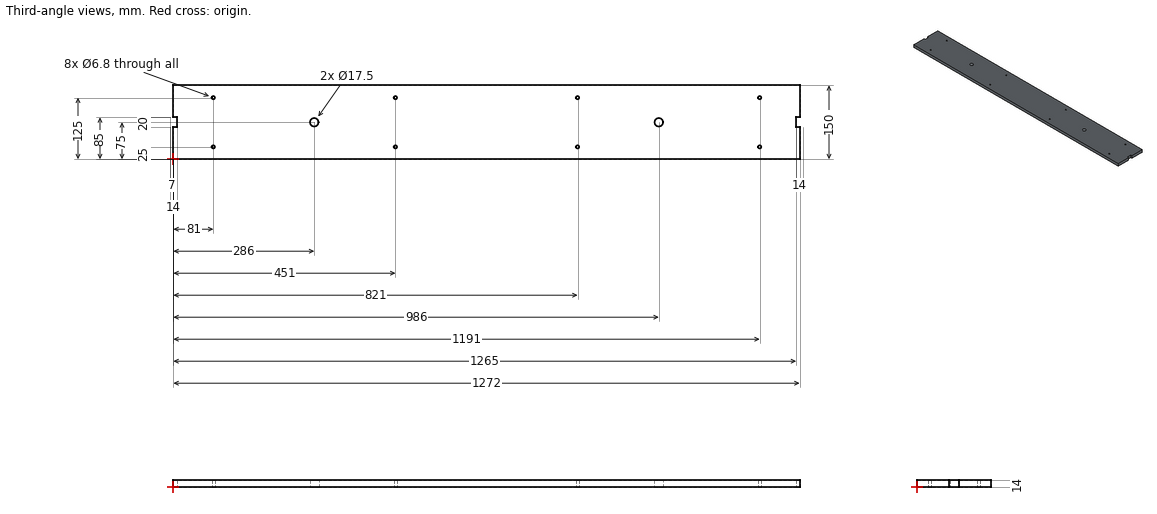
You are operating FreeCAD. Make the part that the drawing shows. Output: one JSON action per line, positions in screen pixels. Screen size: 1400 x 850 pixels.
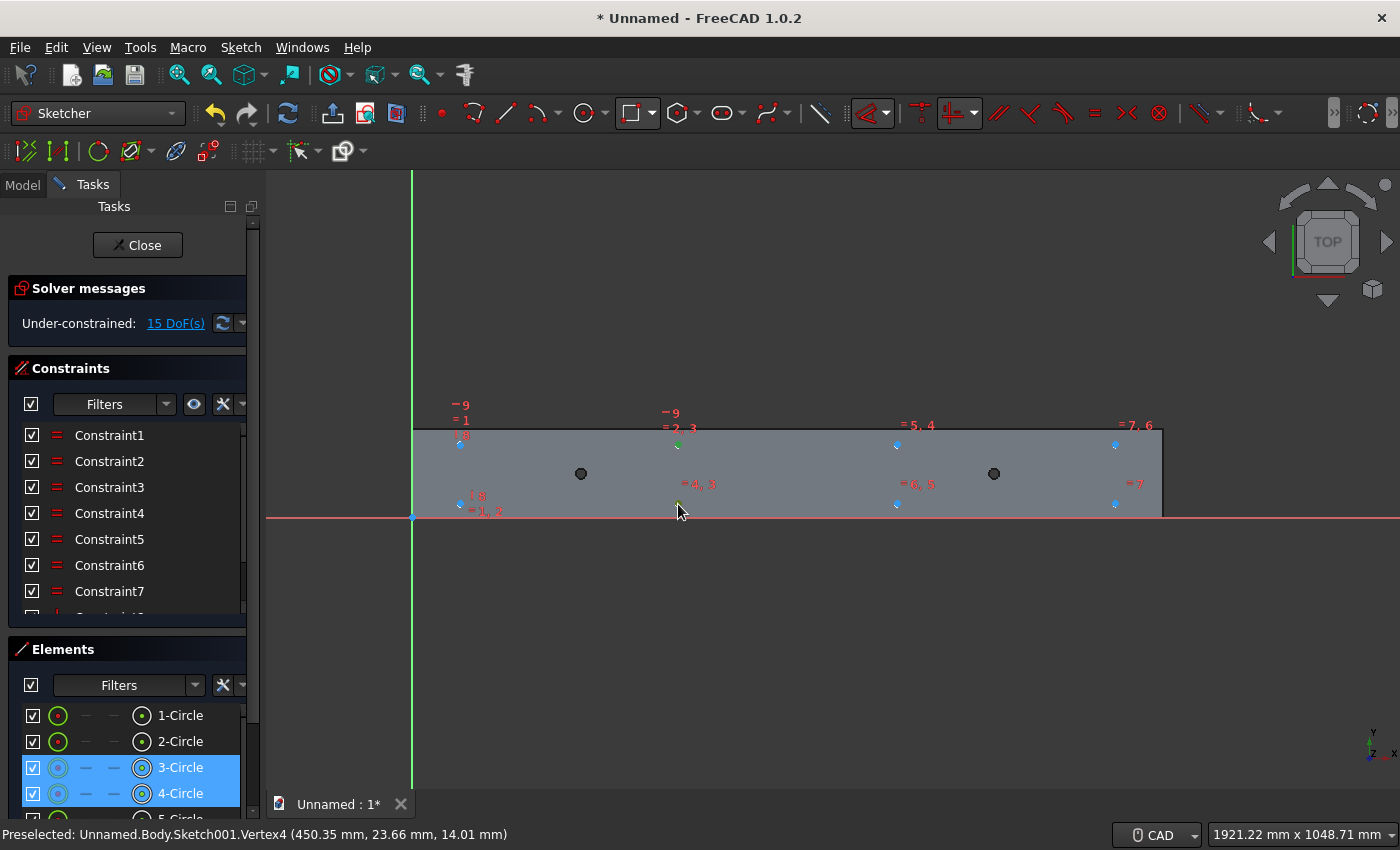
{"action": "left_click", "coordinate": [976, 114]}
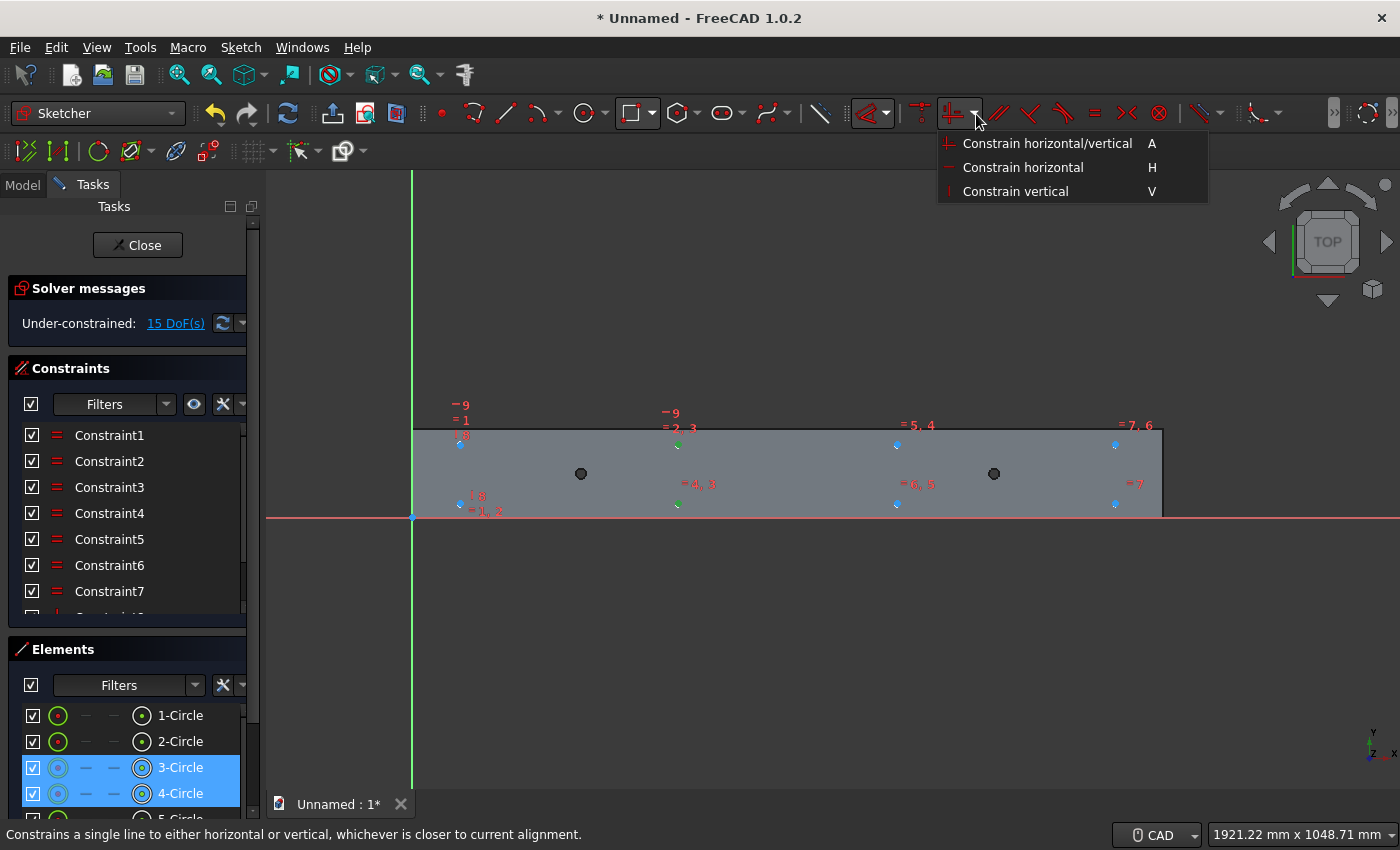
{"action": "left_click", "coordinate": [1073, 191]}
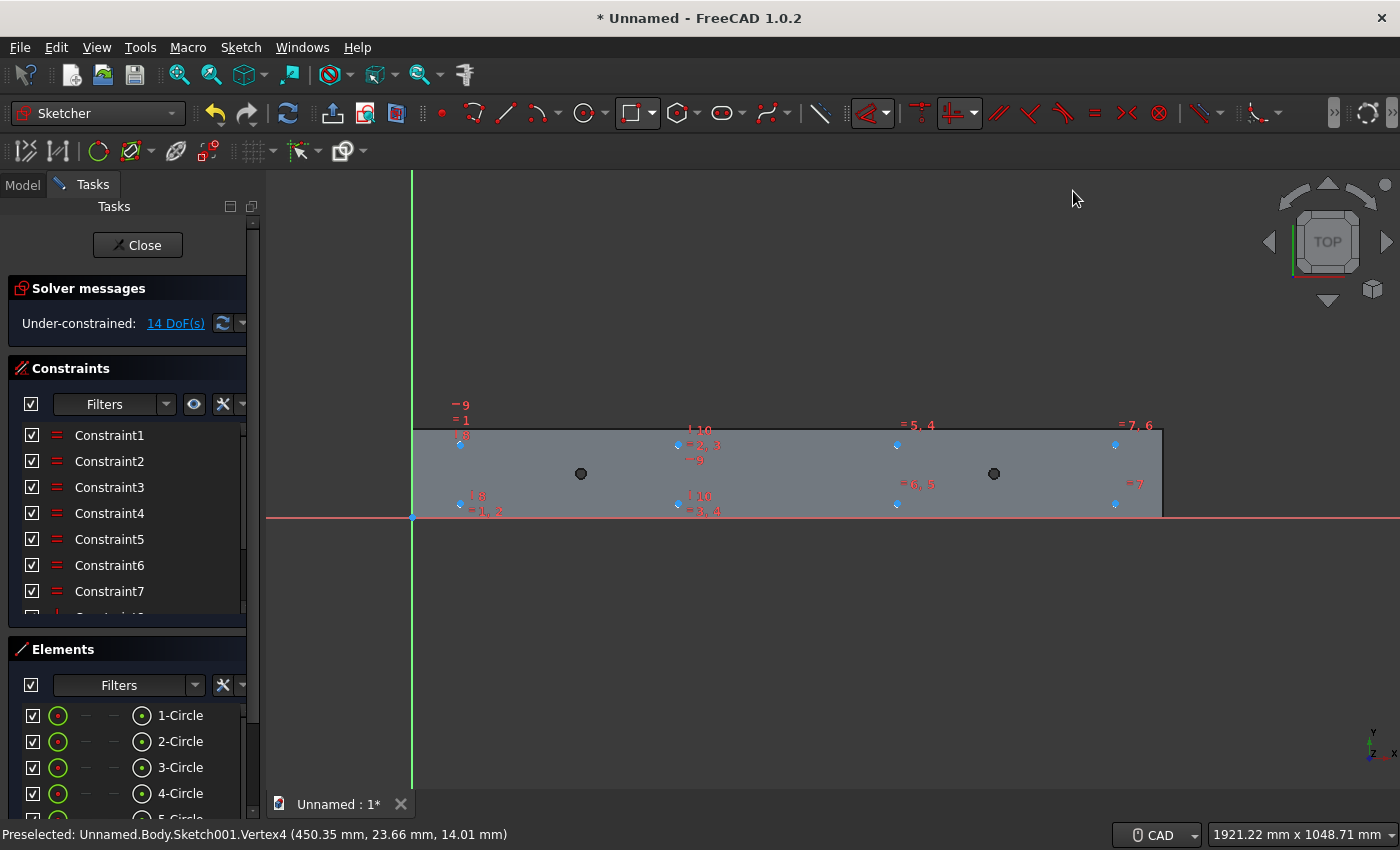
{"action": "left_click", "coordinate": [460, 504]}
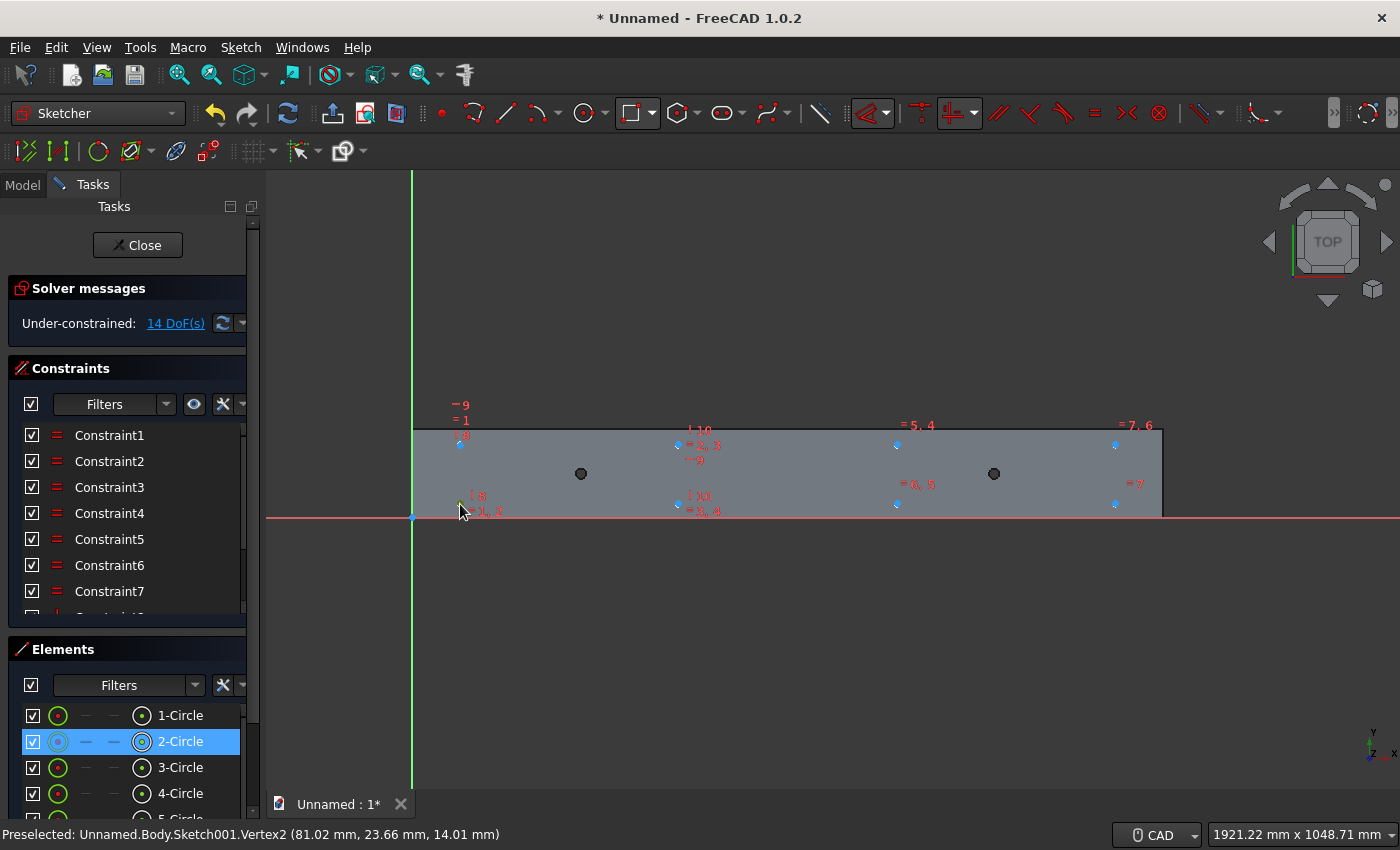
{"action": "left_click", "coordinate": [678, 504]}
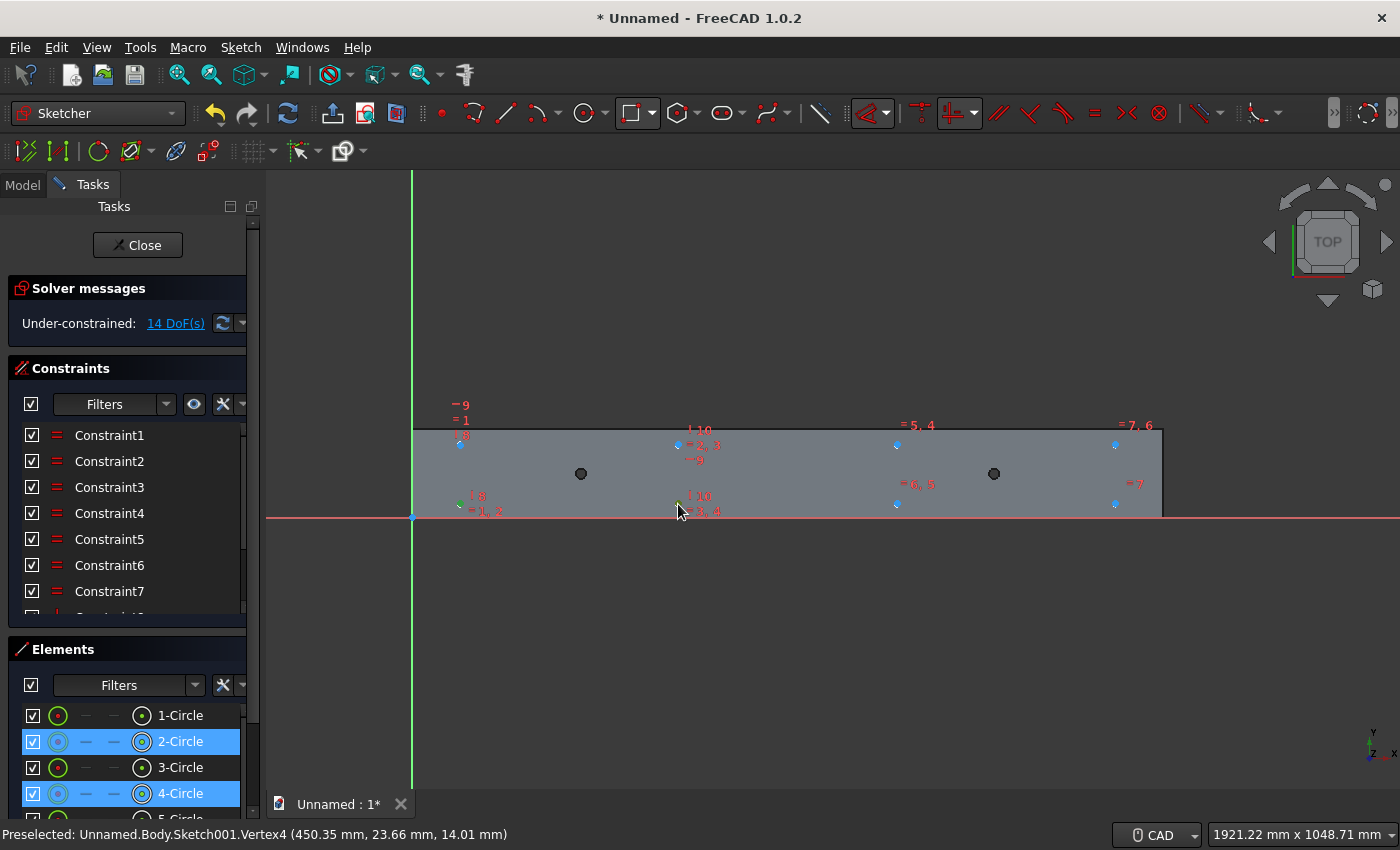
{"action": "key", "text": "h"}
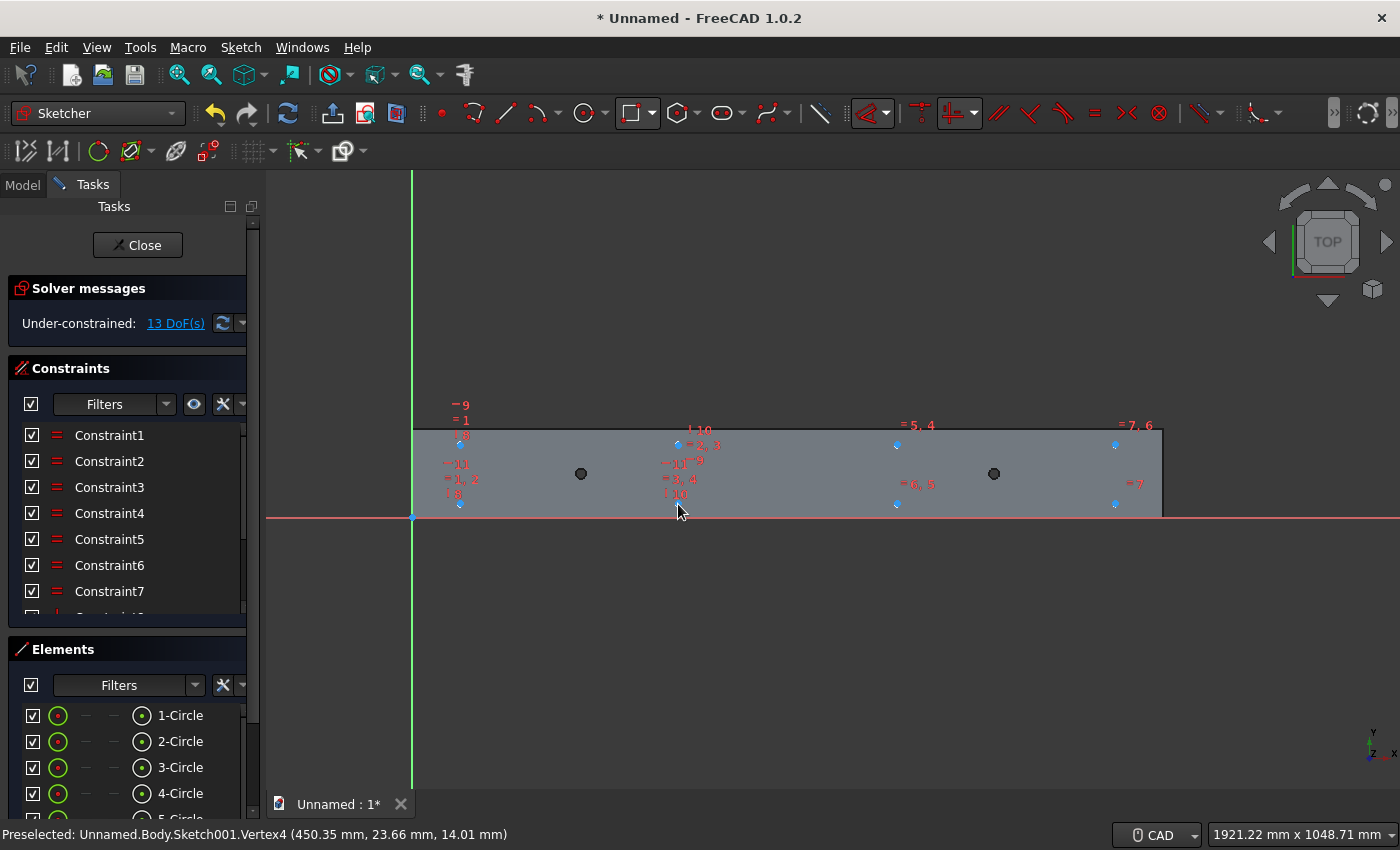
{"action": "left_click", "coordinate": [678, 445]}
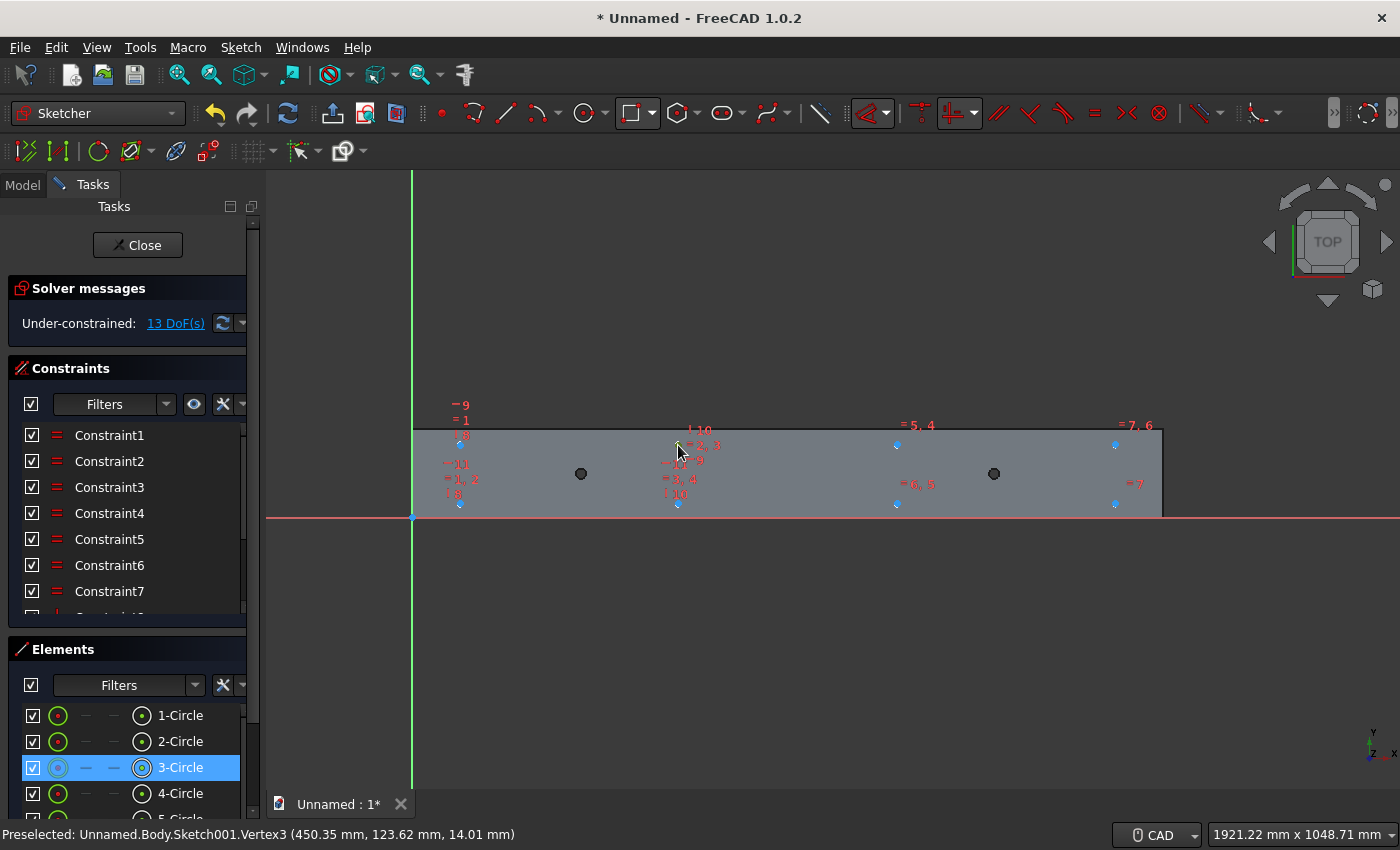
{"action": "left_click", "coordinate": [897, 445]}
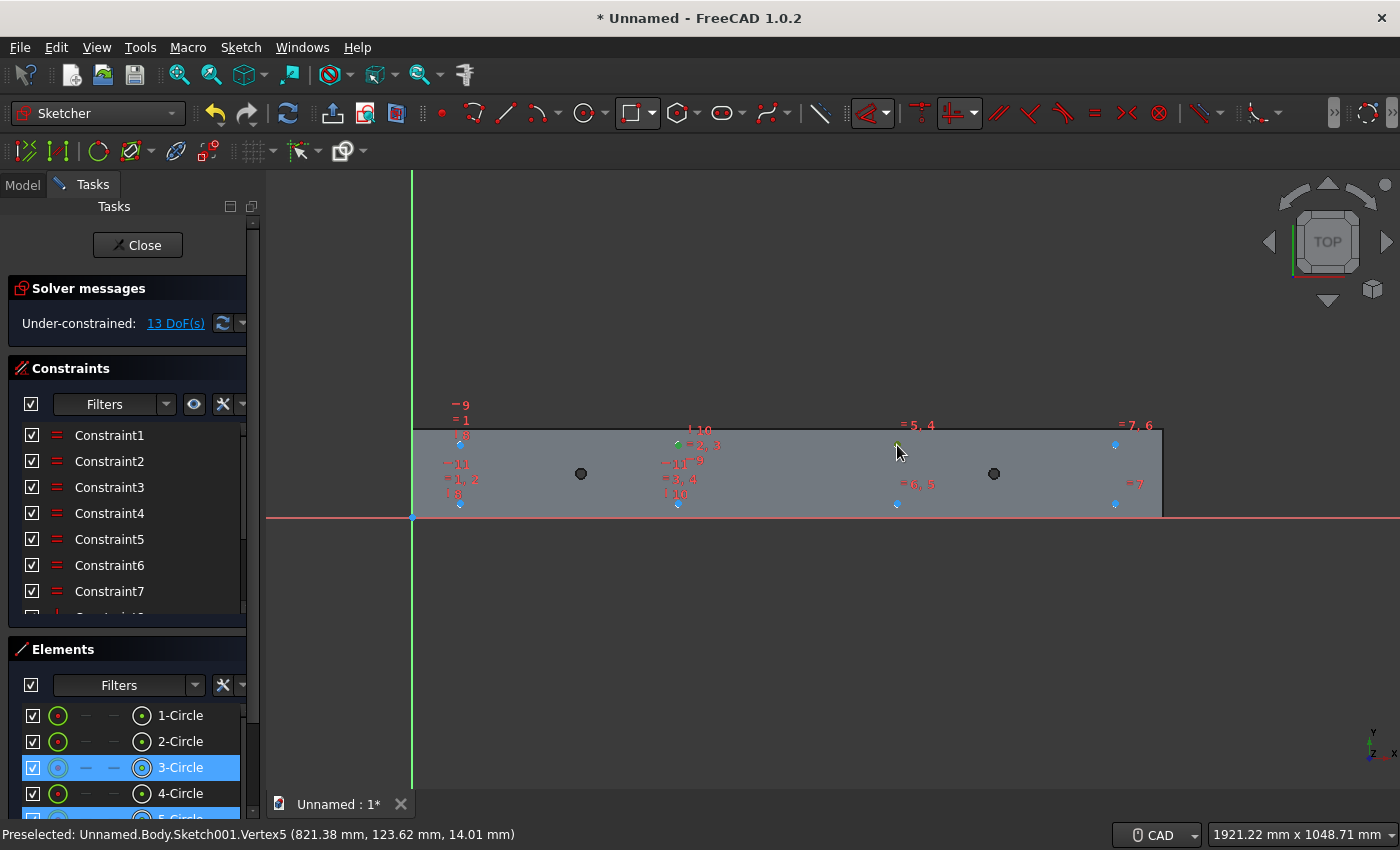
{"action": "left_click", "coordinate": [976, 114]}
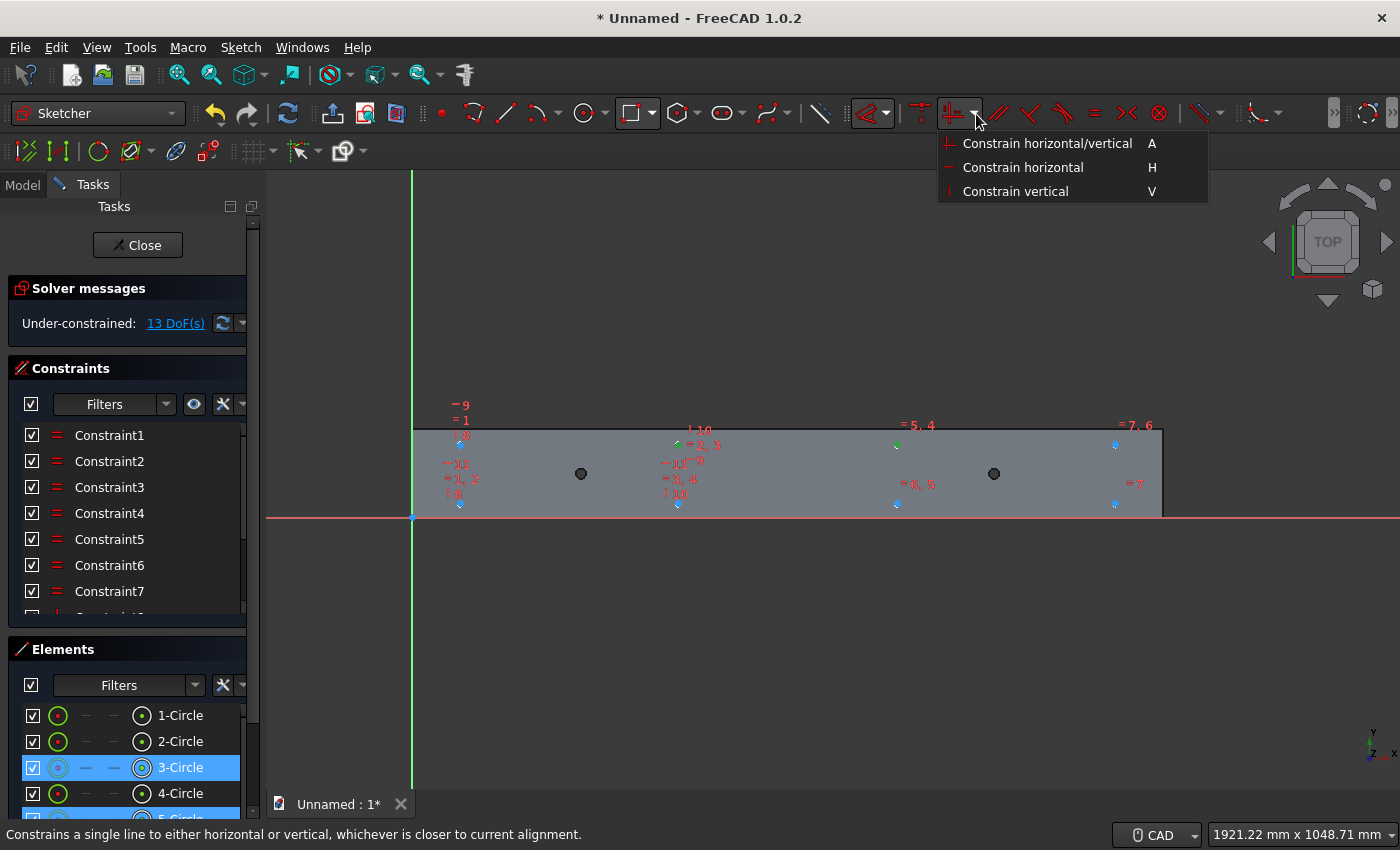
{"action": "left_click", "coordinate": [1073, 167]}